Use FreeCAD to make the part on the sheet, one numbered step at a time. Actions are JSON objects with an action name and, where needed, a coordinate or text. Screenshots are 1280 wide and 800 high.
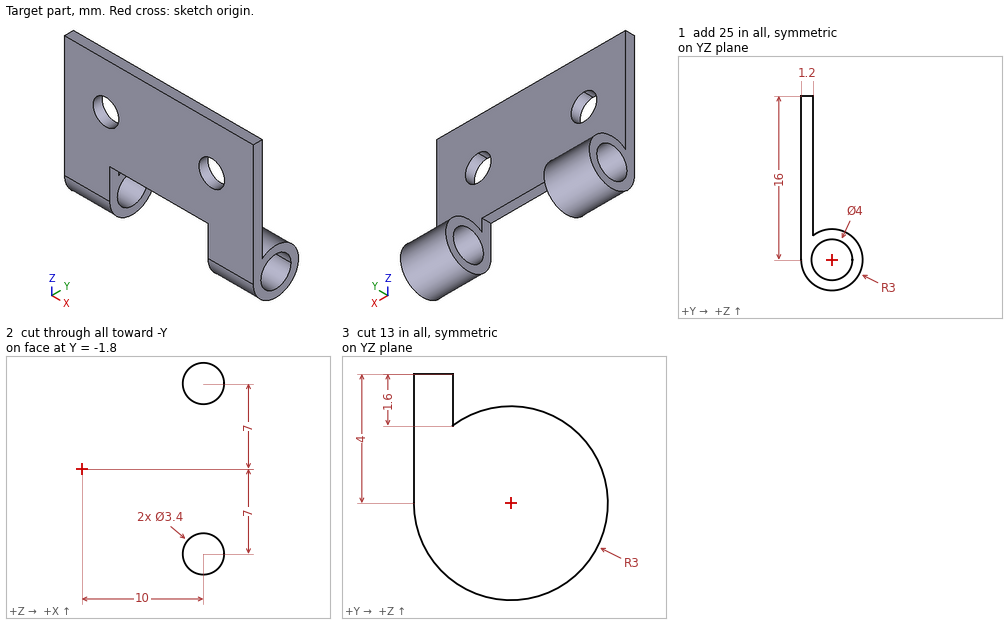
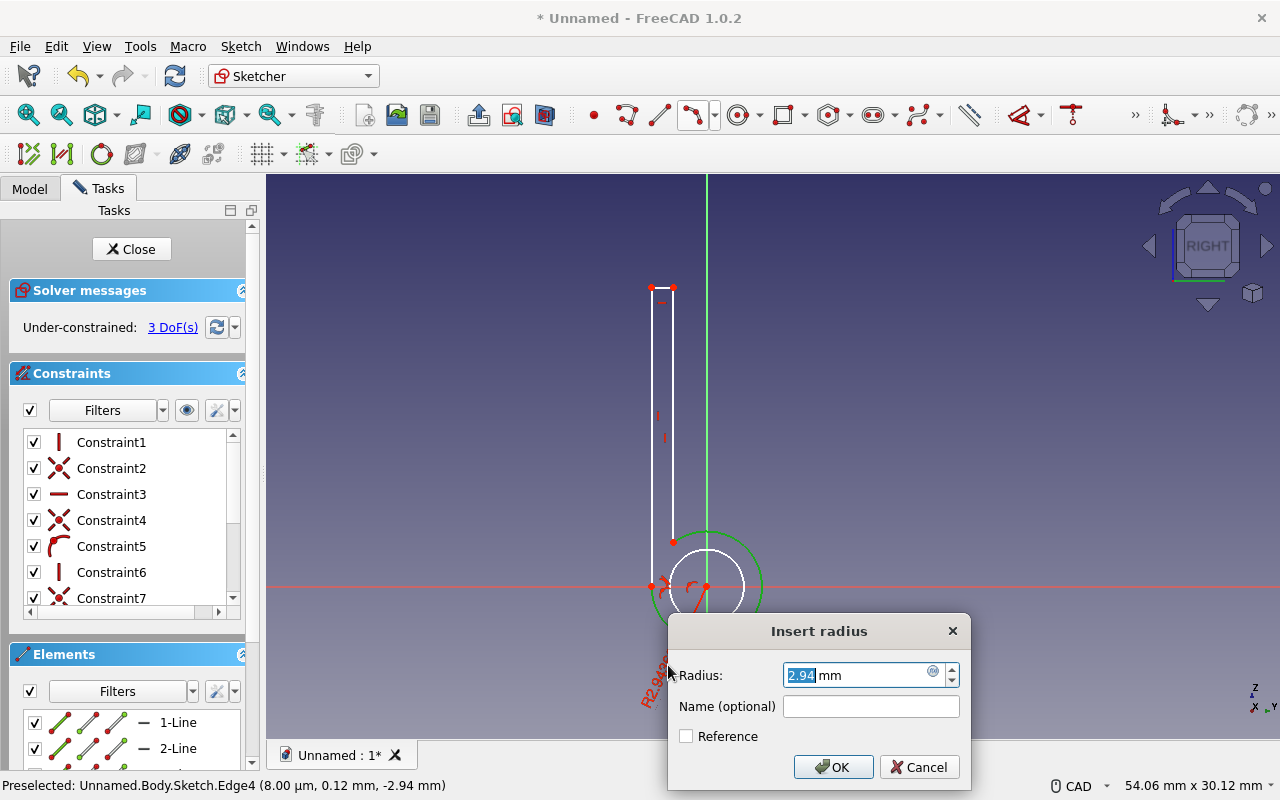
{"action": "type", "text": "3"}
{"action": "key", "text": "Return"}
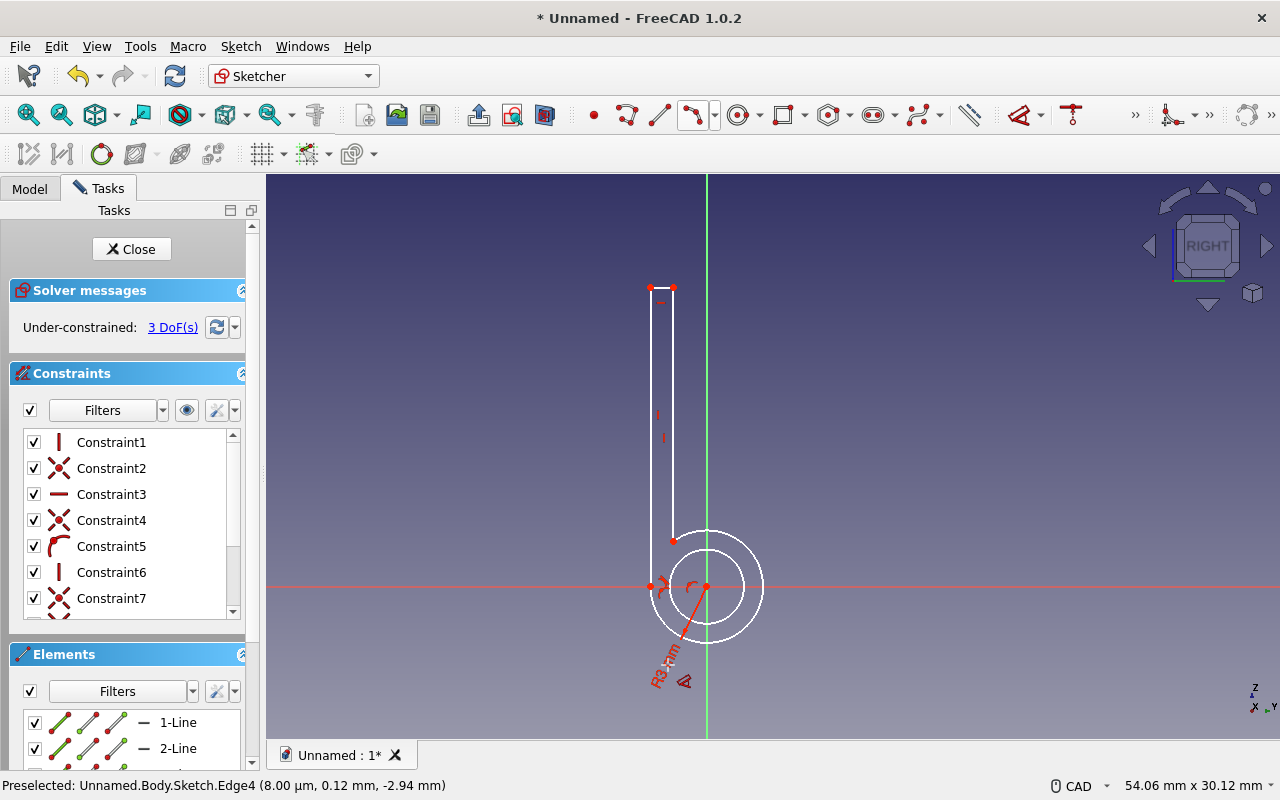
{"action": "left_click", "coordinate": [733, 560]}
{"action": "left_click", "coordinate": [755, 537]}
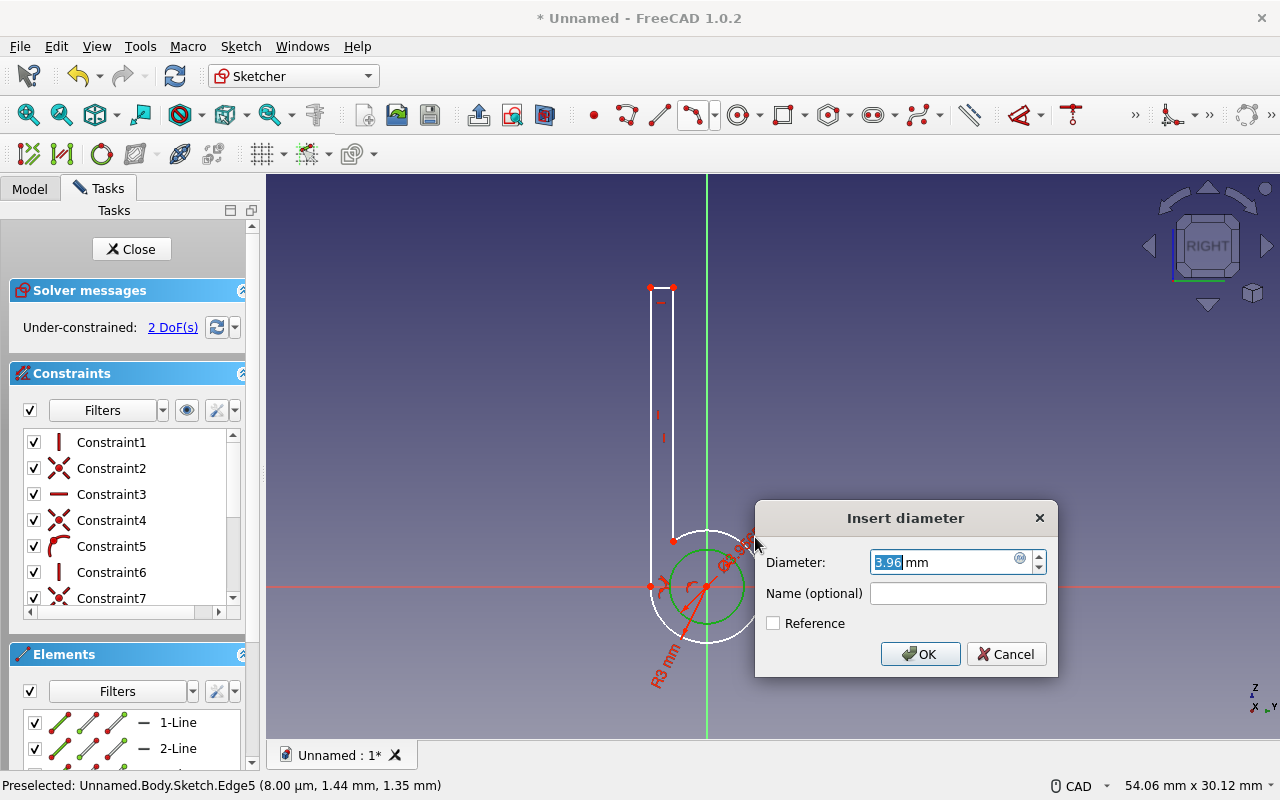
{"action": "type", "text": "4"}
{"action": "key", "text": "Return"}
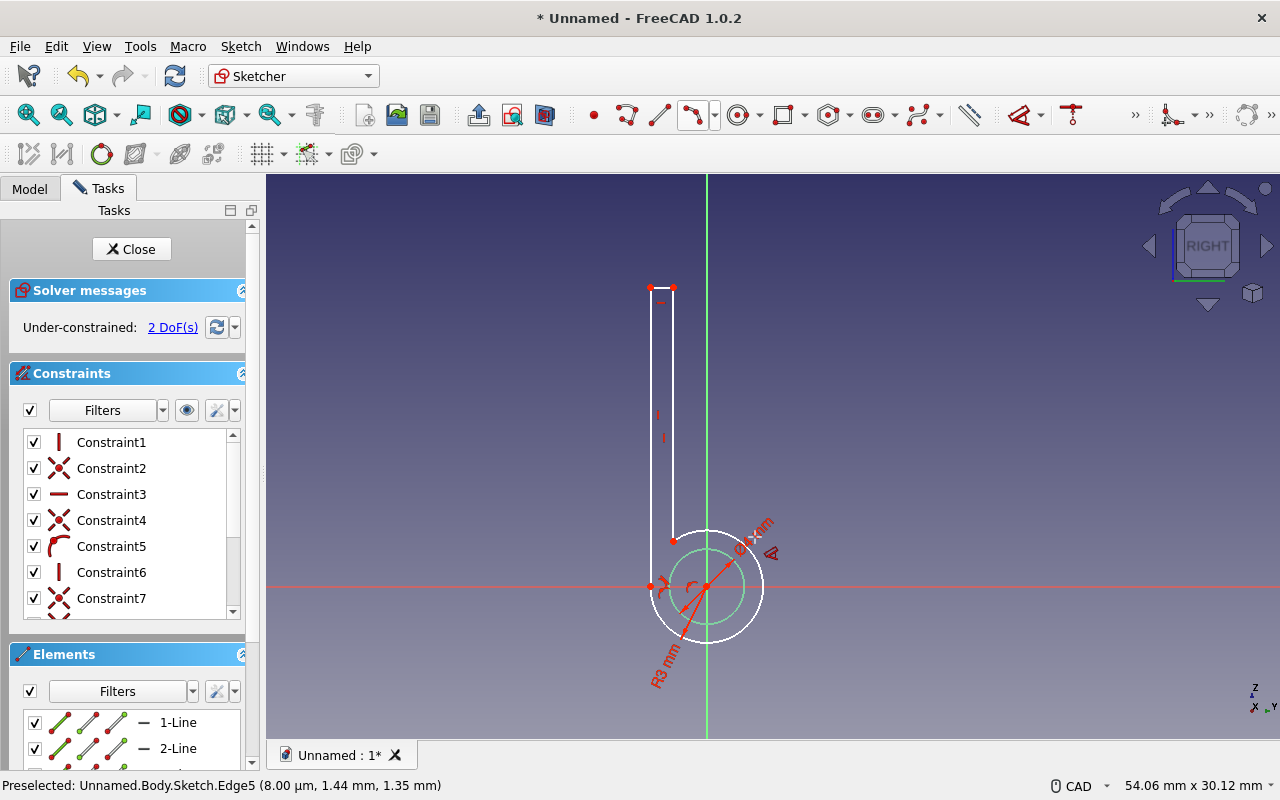
{"action": "left_click", "coordinate": [651, 378]}
{"action": "left_click", "coordinate": [617, 437]}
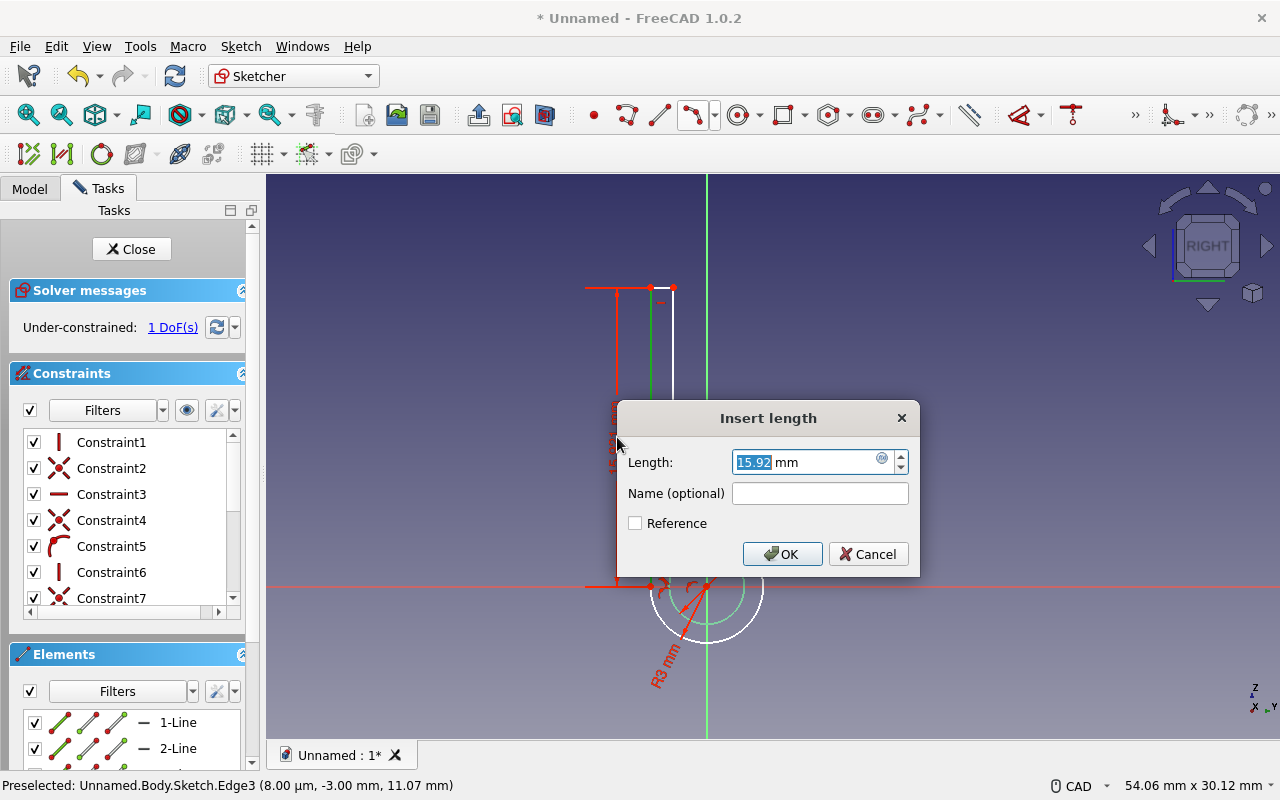
{"action": "type", "text": "16"}
{"action": "key", "text": "Return"}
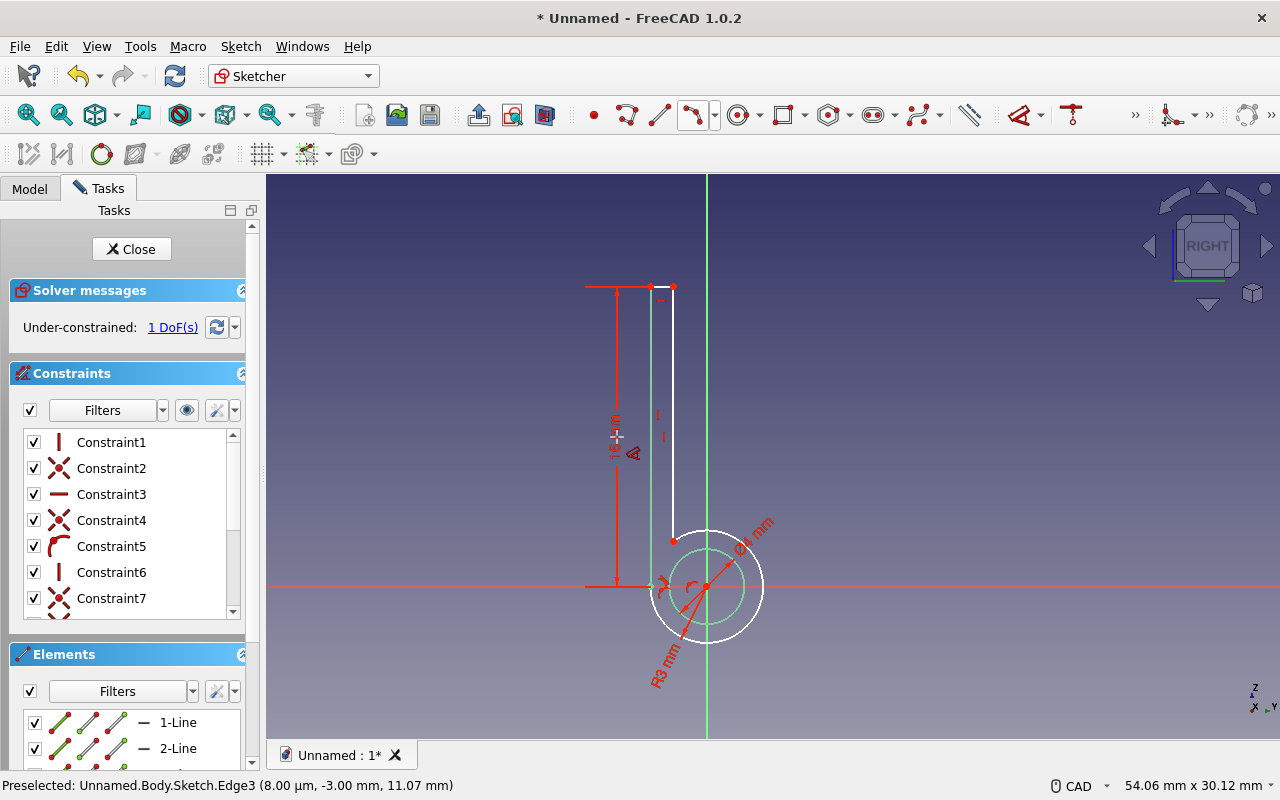
{"action": "scroll", "coordinate": [662, 287], "scroll_direction": "up", "scroll_amount": 3}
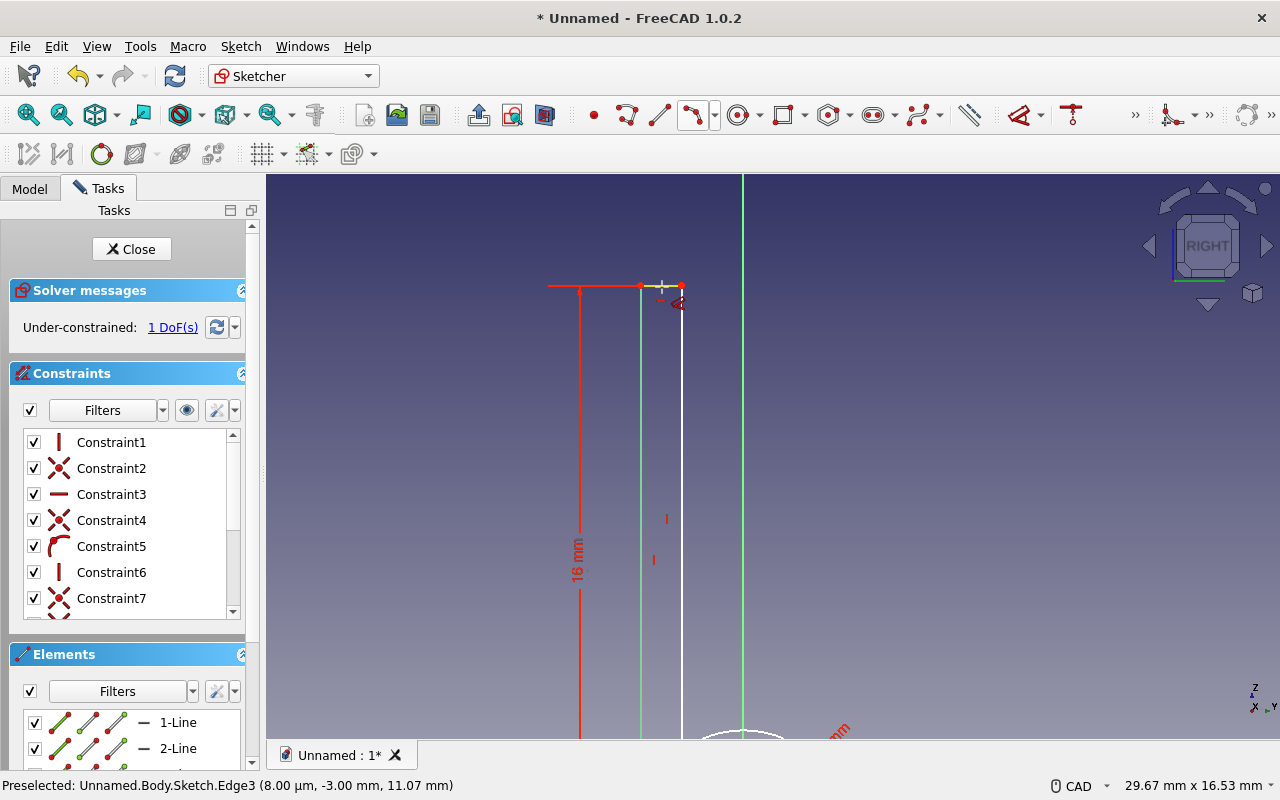
{"action": "left_click", "coordinate": [661, 286]}
{"action": "left_click", "coordinate": [661, 252]}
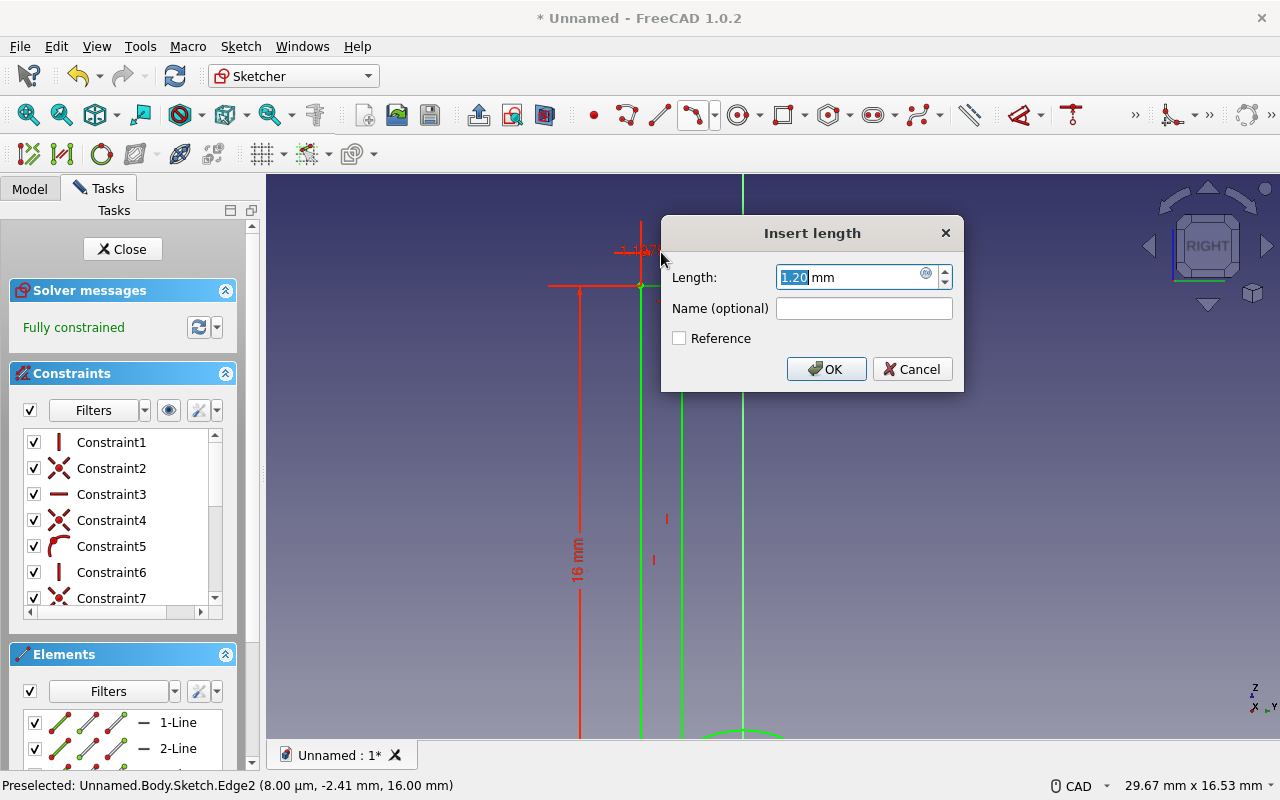
{"action": "type", "text": "1.2"}
{"action": "key", "text": "Return"}
{"action": "key", "text": "Escape"}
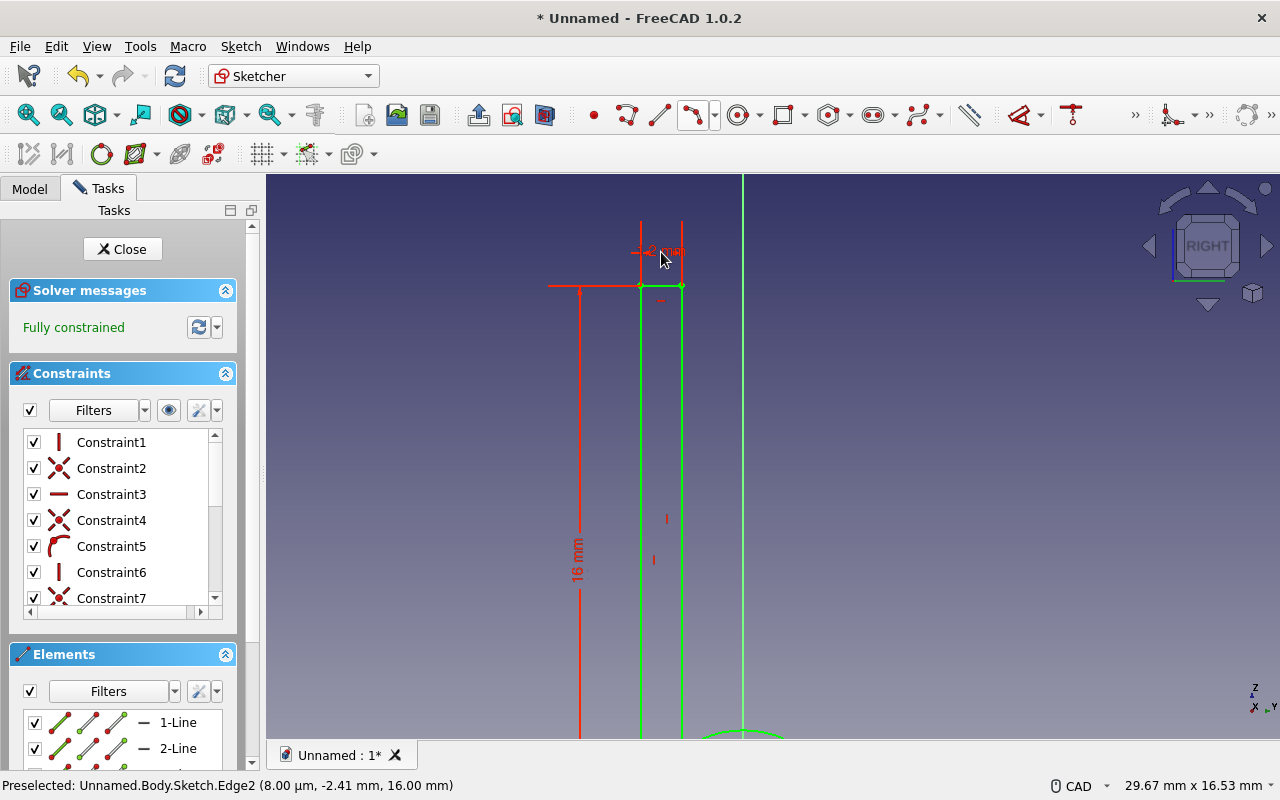
{"action": "left_click", "coordinate": [123, 249]}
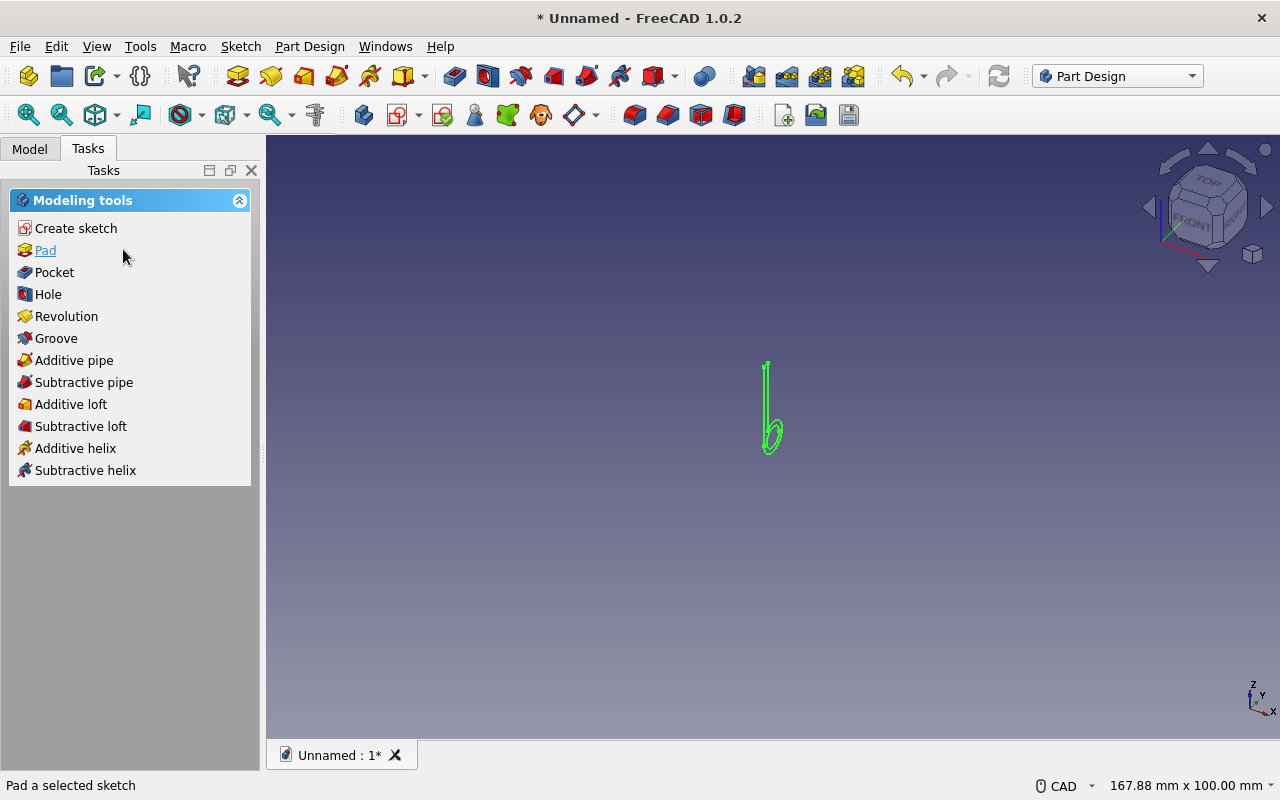
{"action": "left_click", "coordinate": [238, 76]}